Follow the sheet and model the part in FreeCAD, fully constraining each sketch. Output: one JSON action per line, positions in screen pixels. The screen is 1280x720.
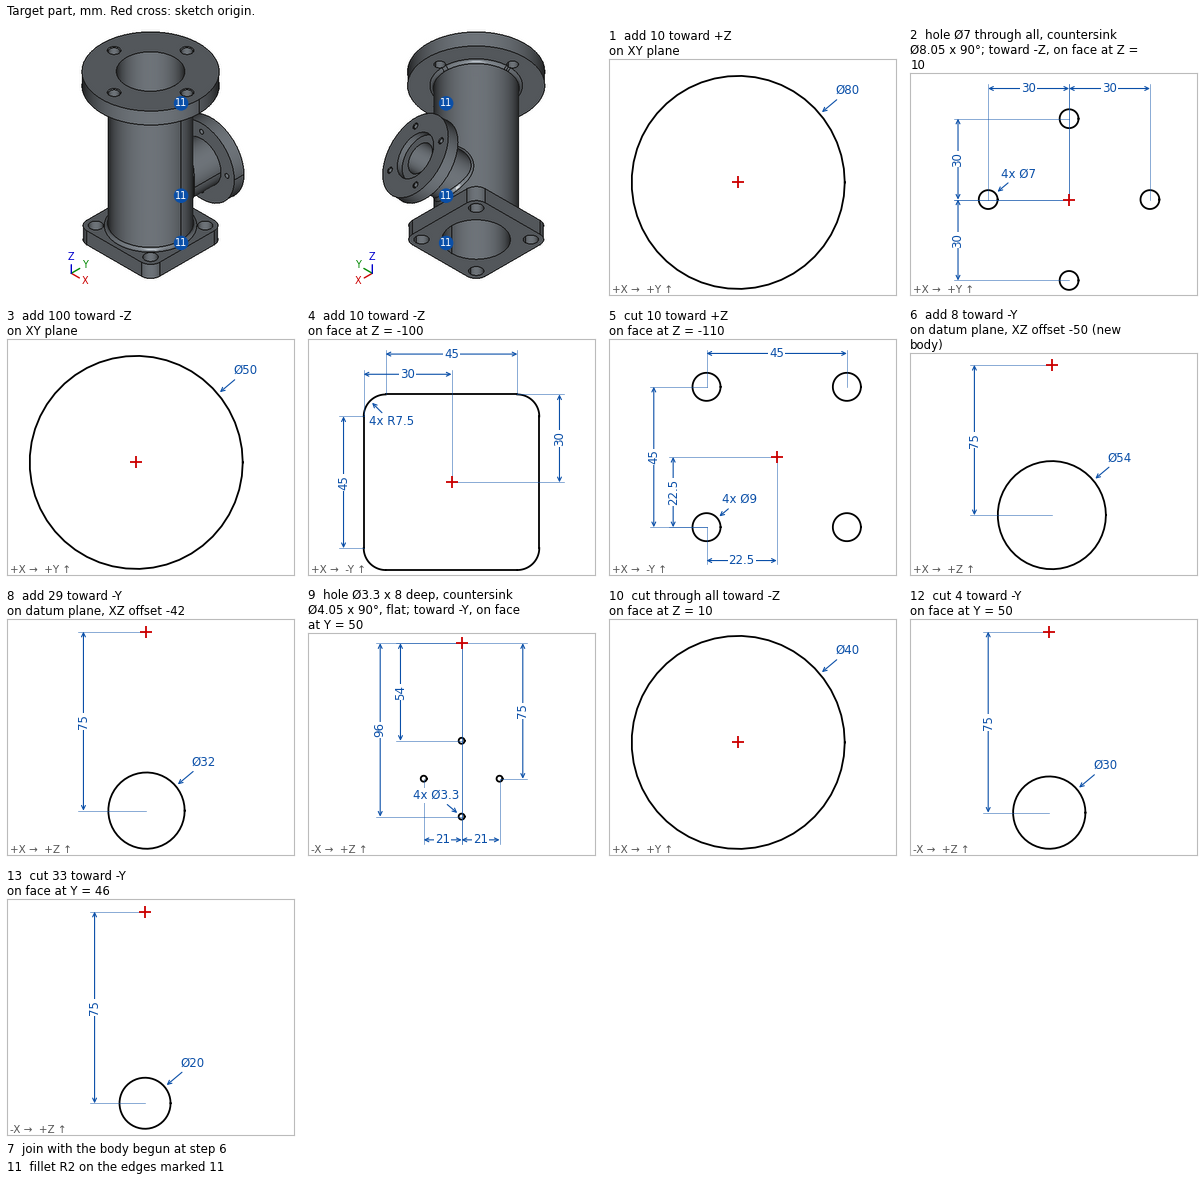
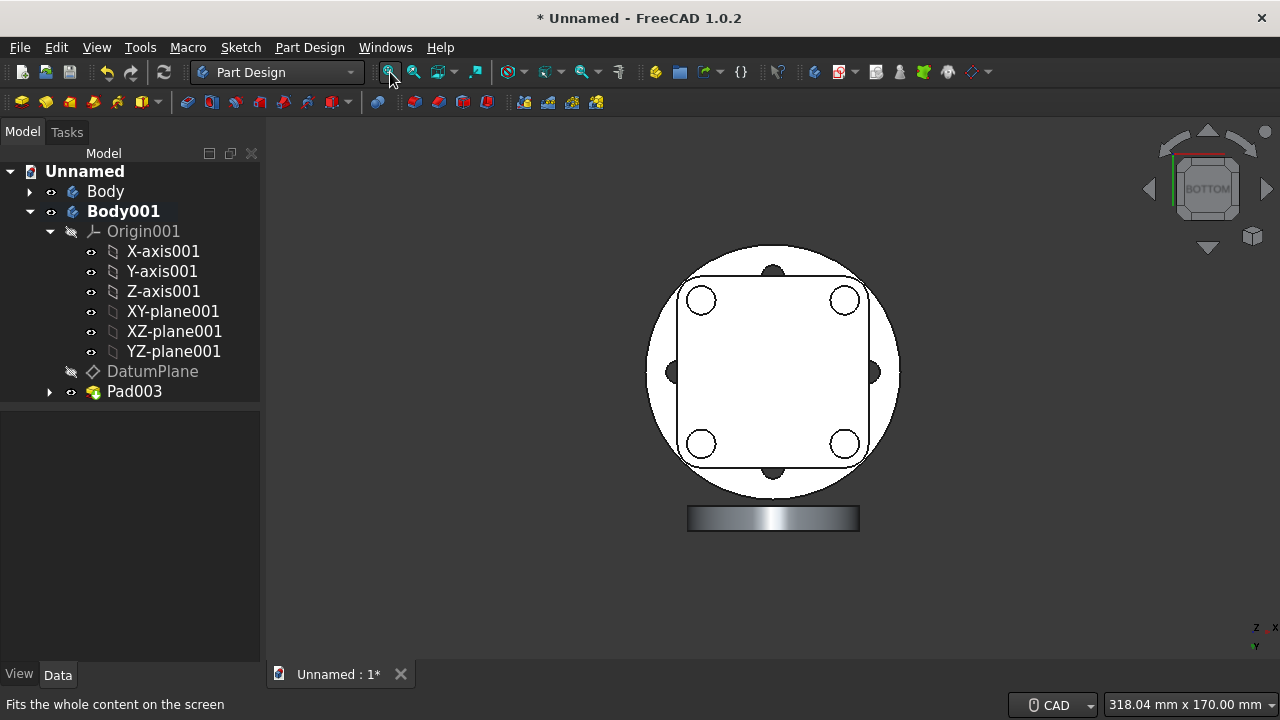
{"action": "double_click", "coordinate": [96, 192]}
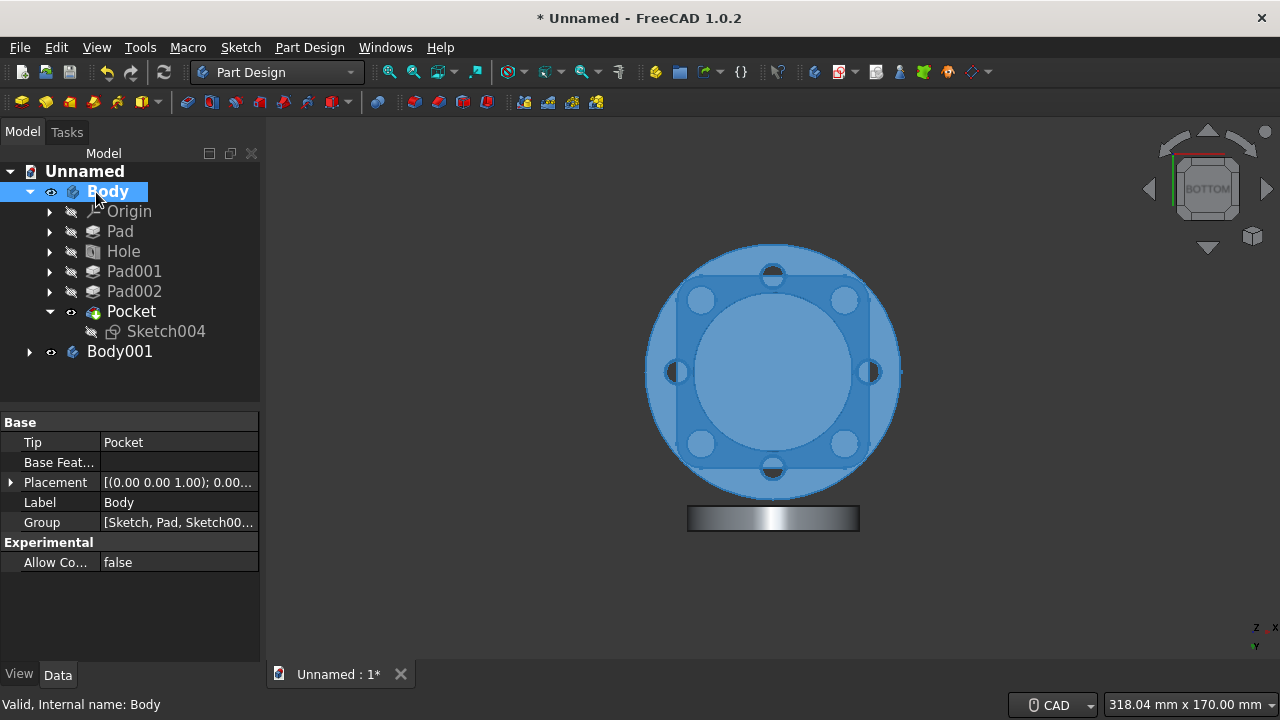
{"action": "left_click", "coordinate": [96, 192]}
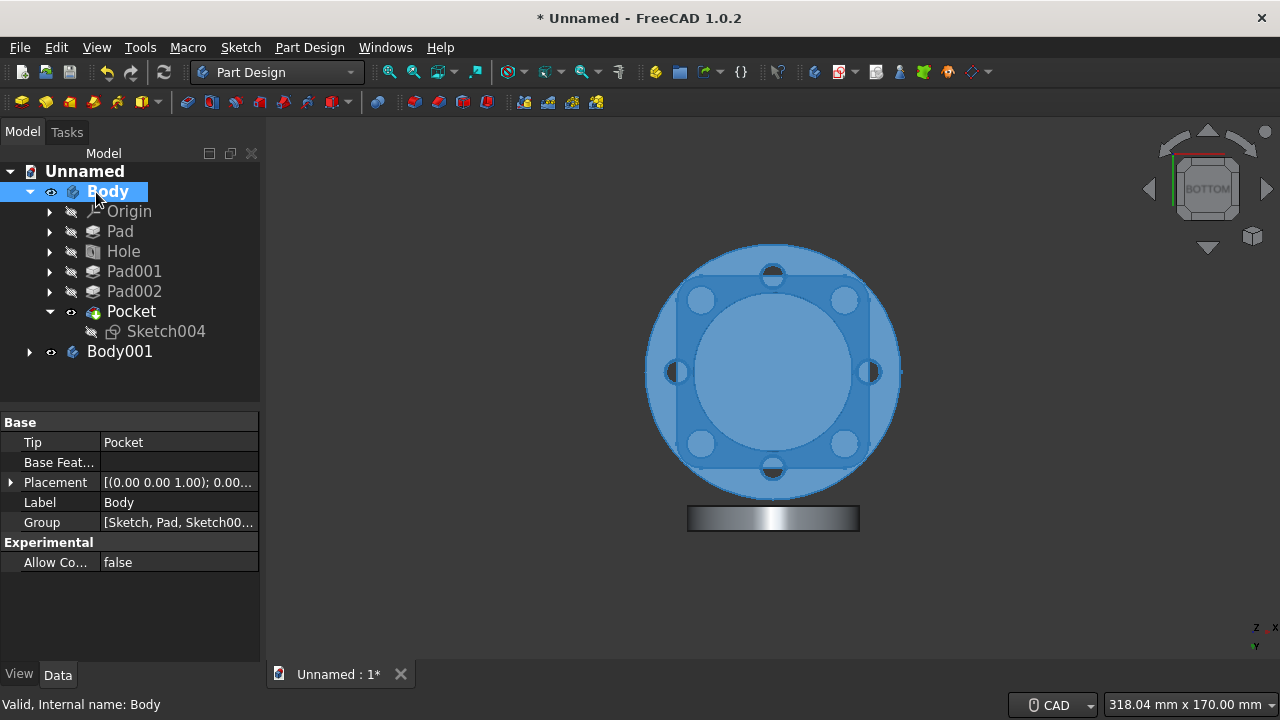
{"action": "left_click", "coordinate": [146, 562]}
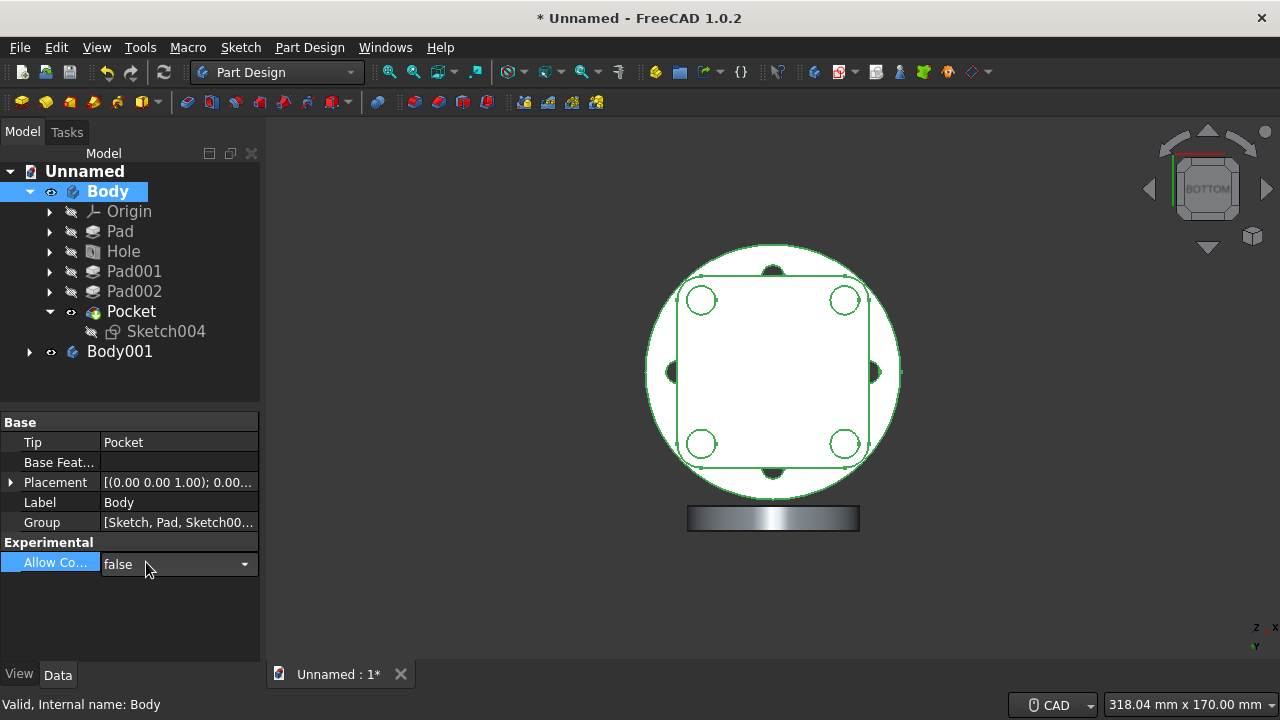
{"action": "left_click", "coordinate": [146, 562]}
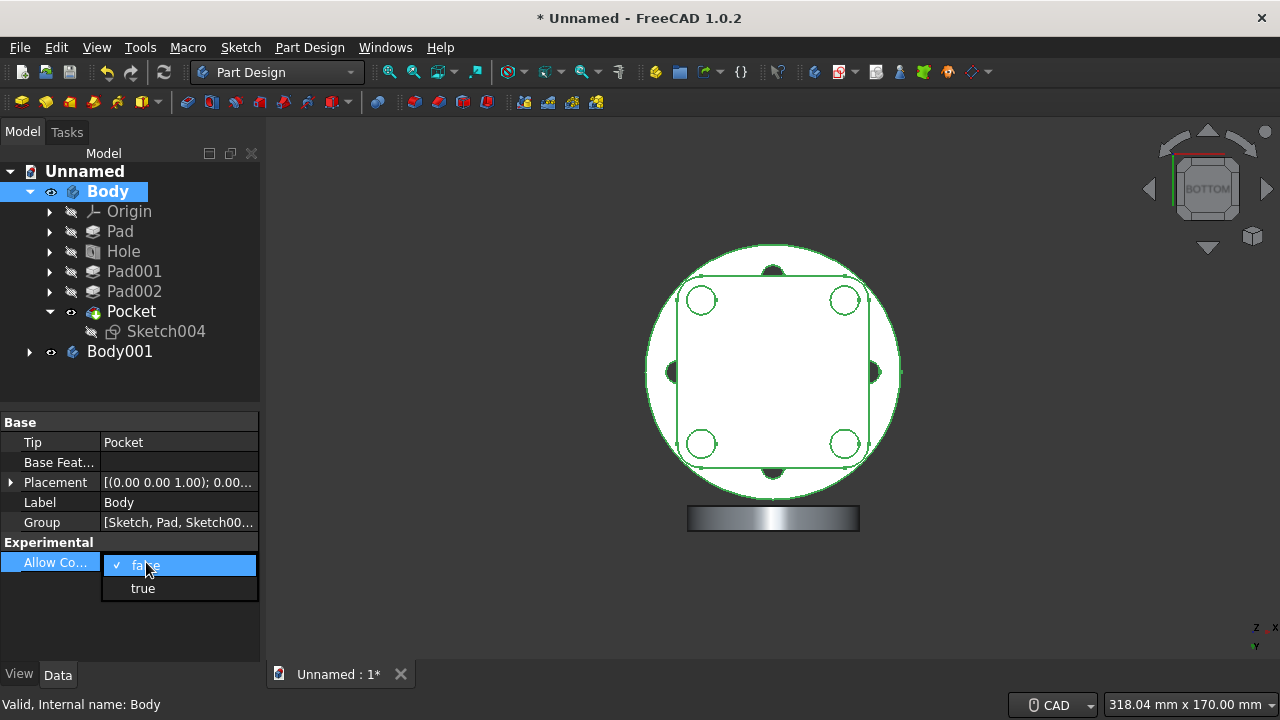
{"action": "left_click", "coordinate": [179, 588]}
{"action": "key", "text": "Return"}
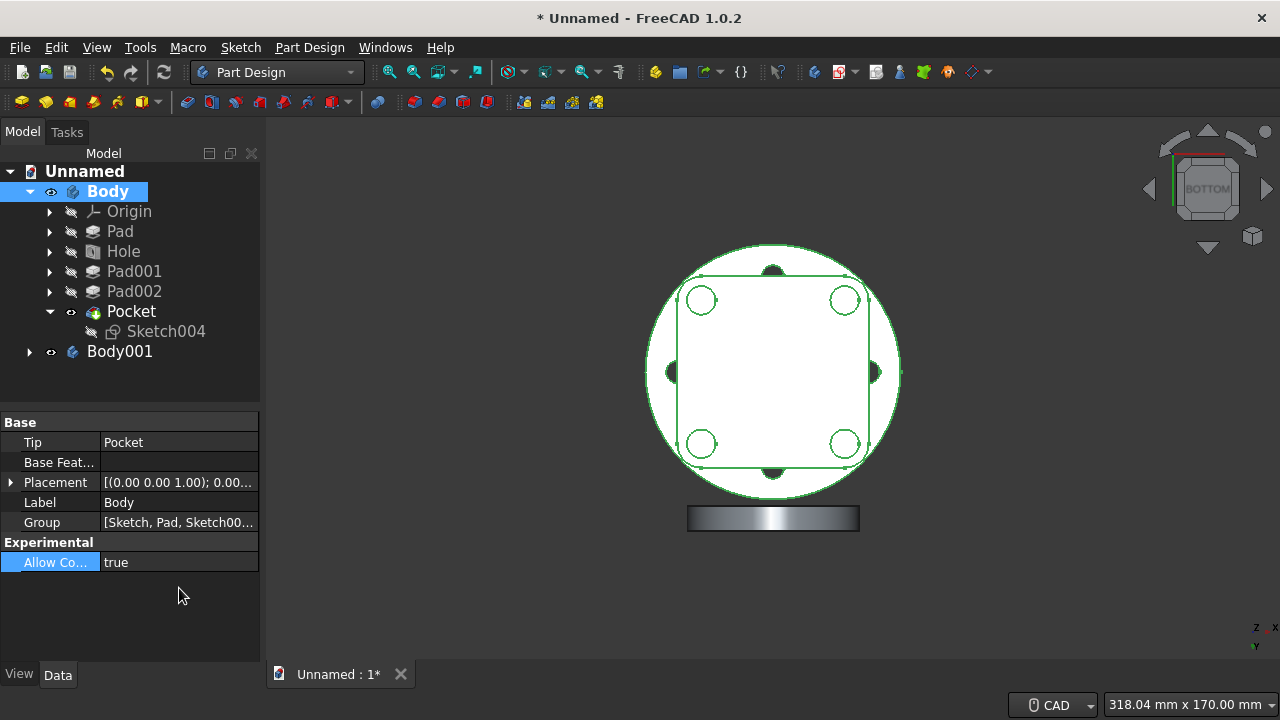
{"action": "left_click", "coordinate": [96, 352]}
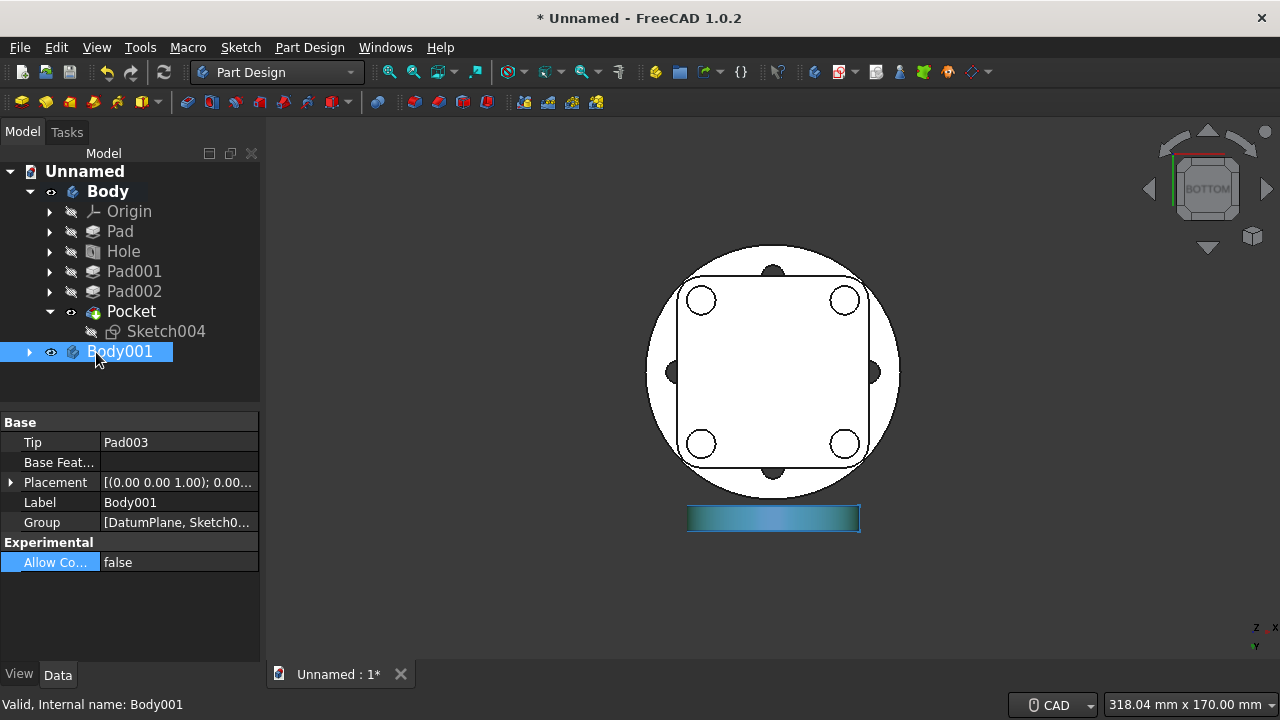
{"action": "left_click", "coordinate": [378, 102]}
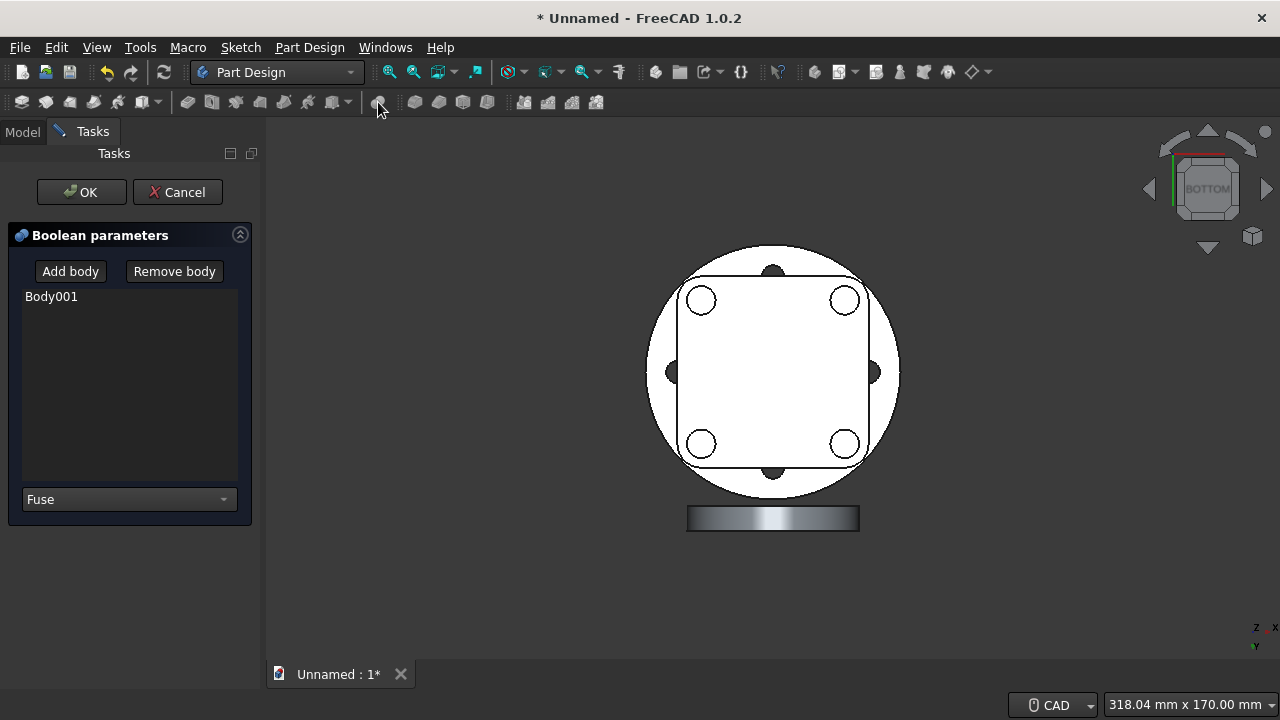
{"action": "left_click", "coordinate": [82, 192]}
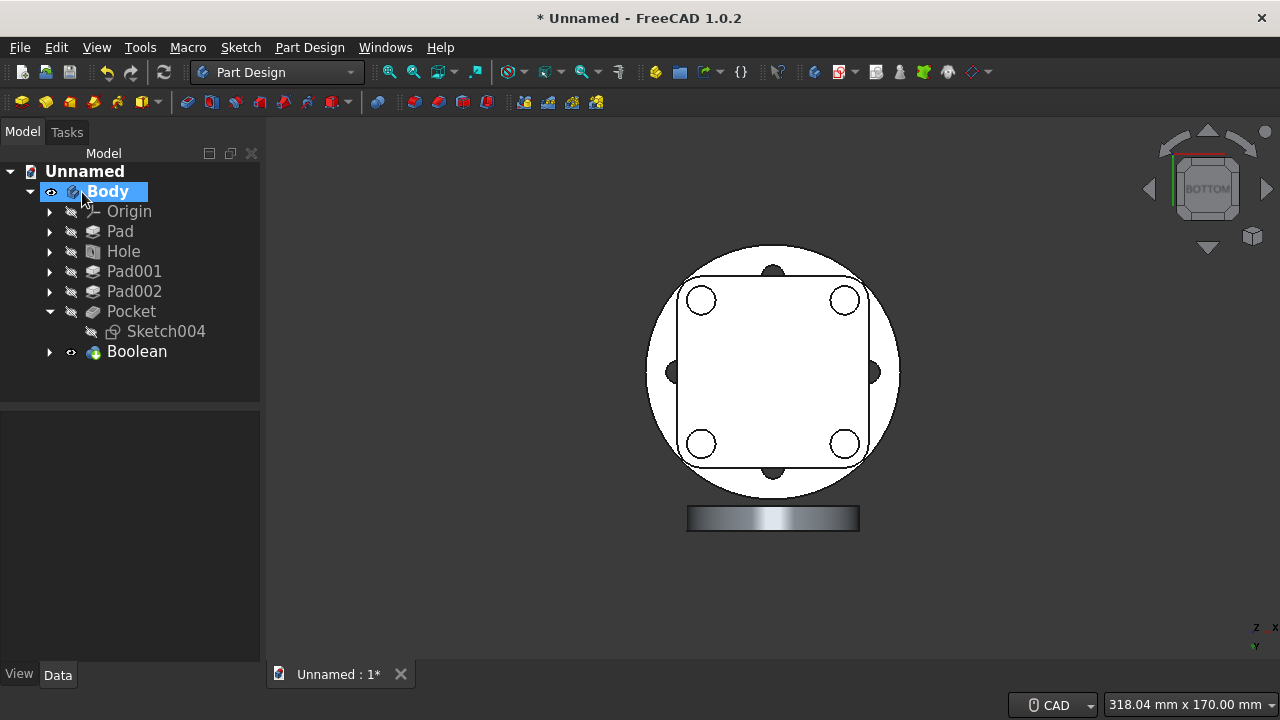
{"action": "left_click", "coordinate": [50, 212]}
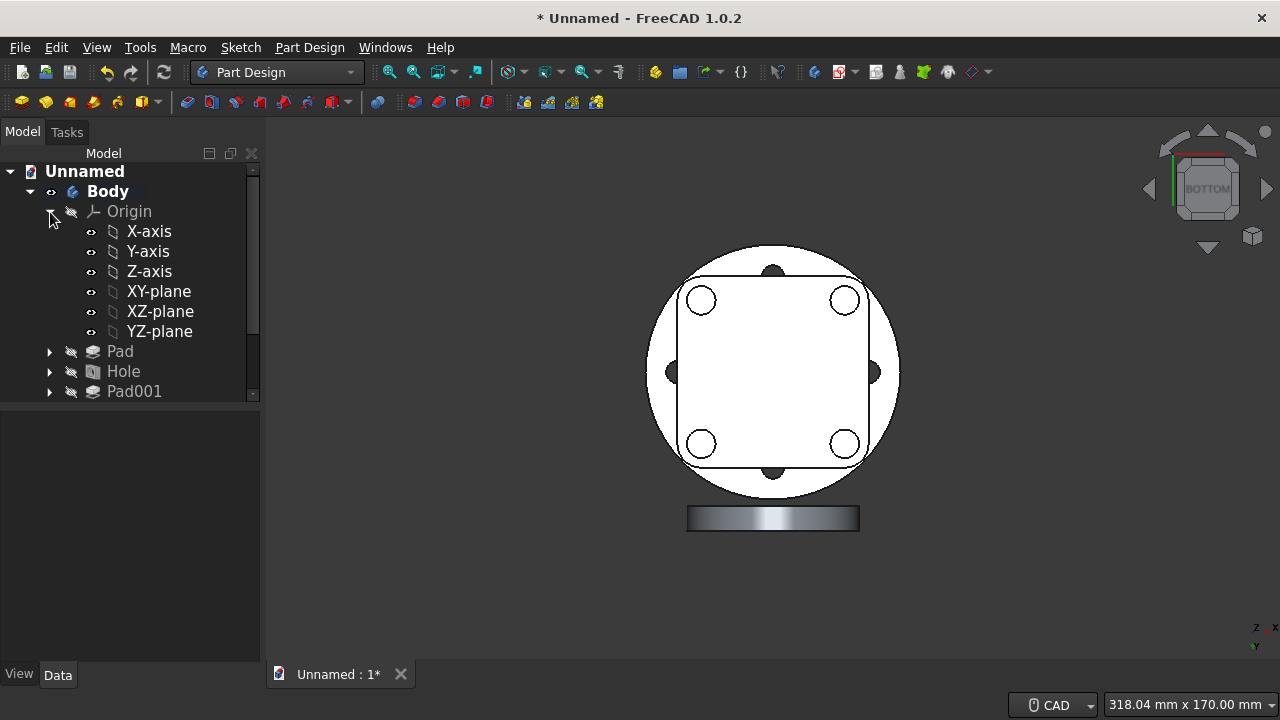
{"action": "left_click", "coordinate": [136, 312]}